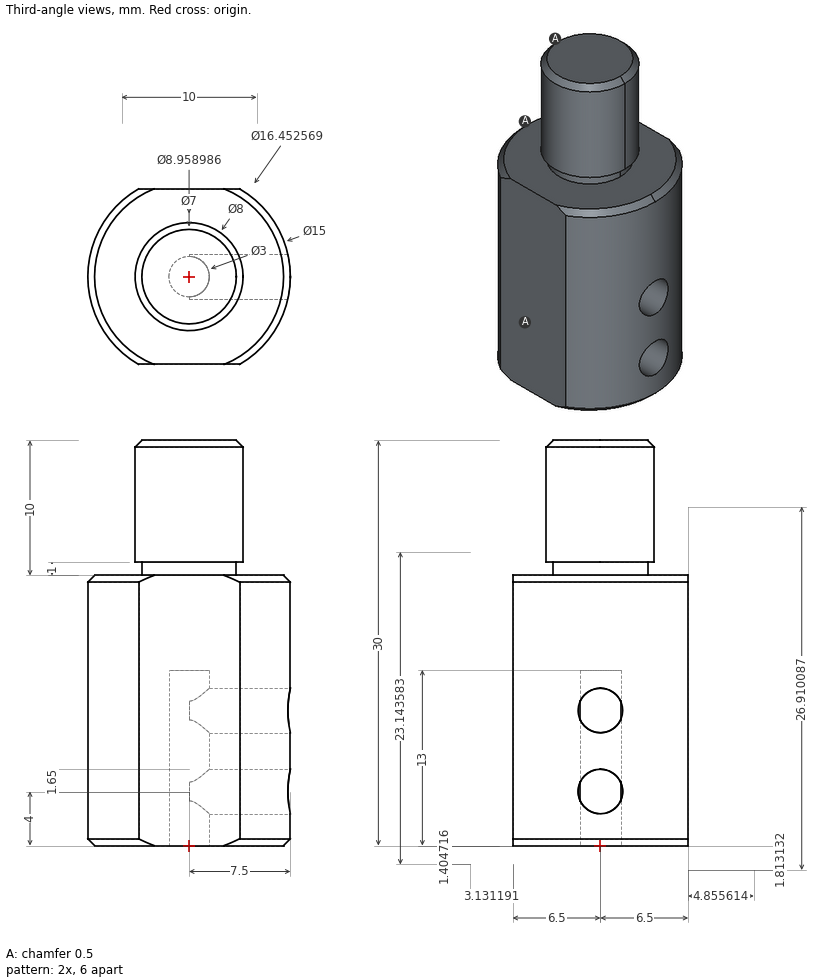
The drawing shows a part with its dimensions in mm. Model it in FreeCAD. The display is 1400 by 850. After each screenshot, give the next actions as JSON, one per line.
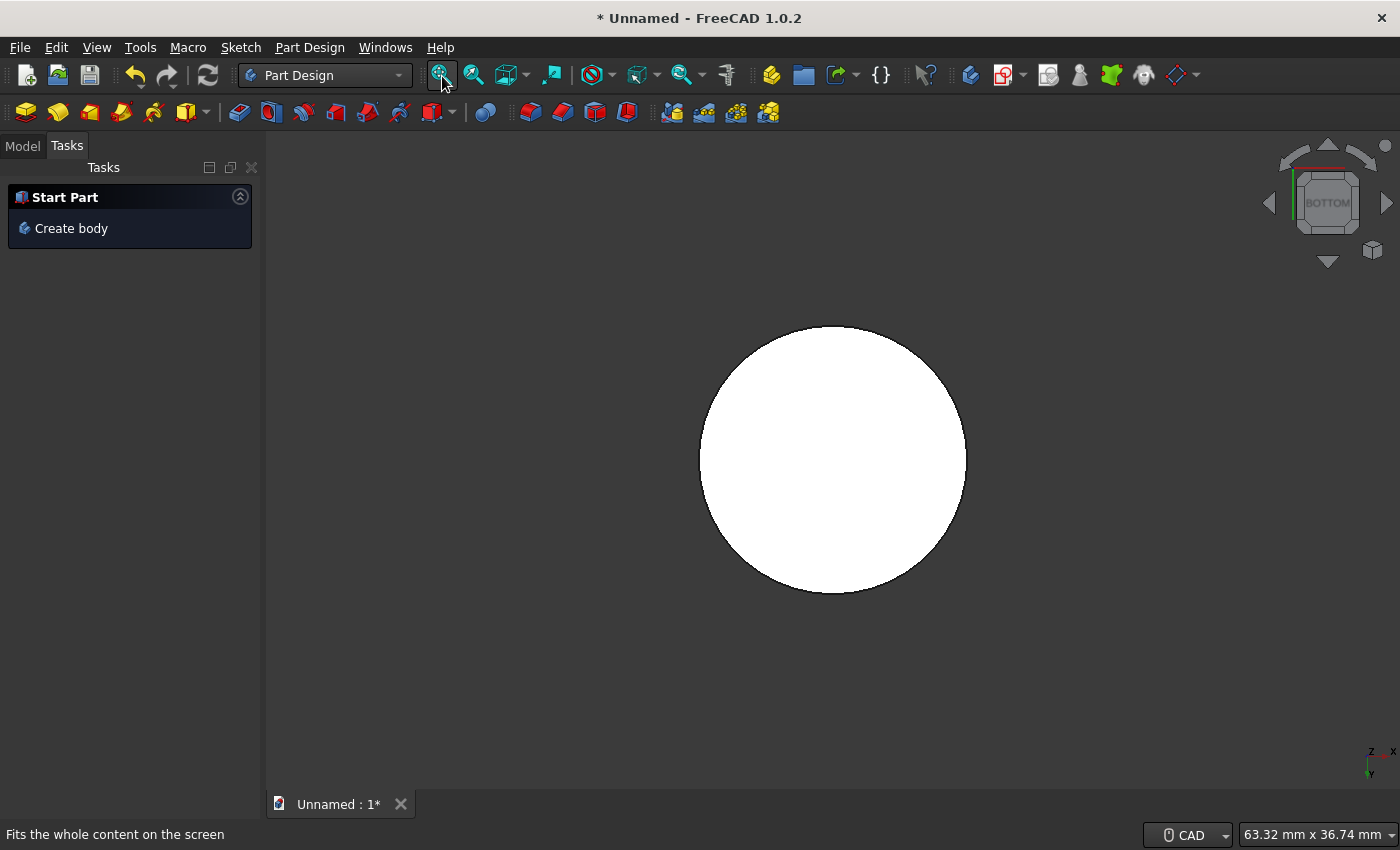
{"action": "left_click", "coordinate": [833, 459]}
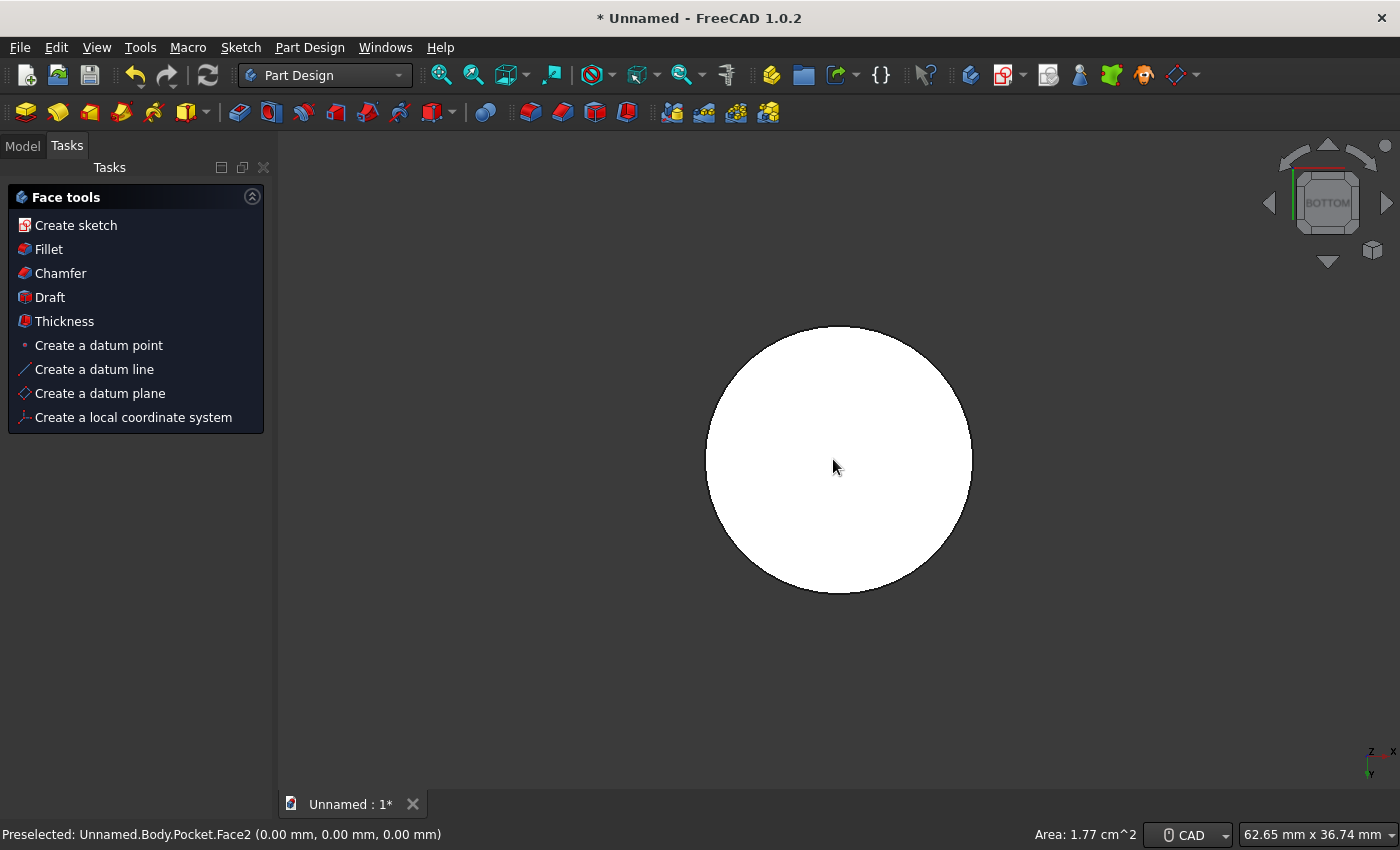
{"action": "left_click", "coordinate": [1004, 76]}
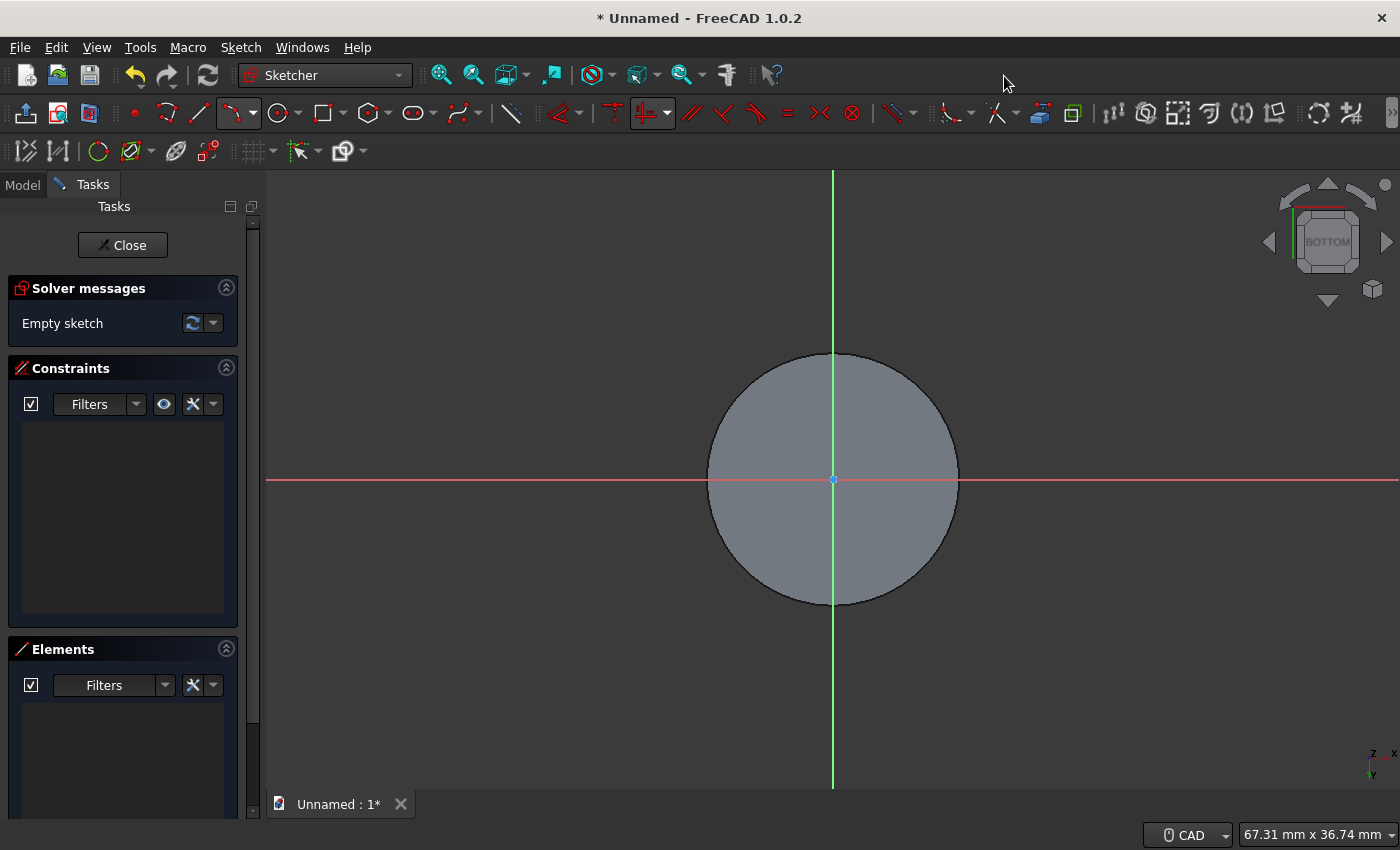
{"action": "scroll", "coordinate": [844, 480], "scroll_direction": "up", "scroll_amount": 10}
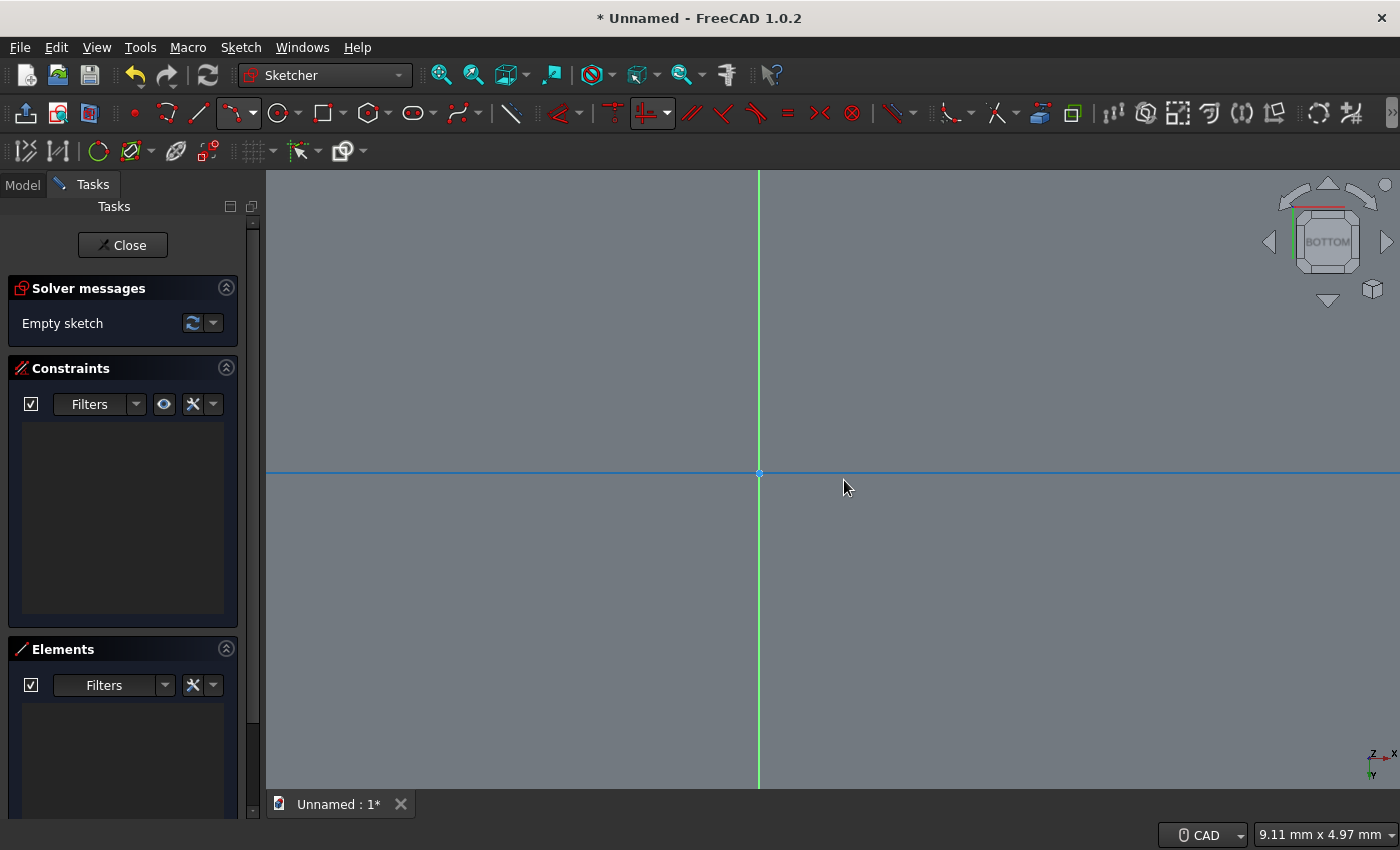
{"action": "left_click", "coordinate": [278, 114]}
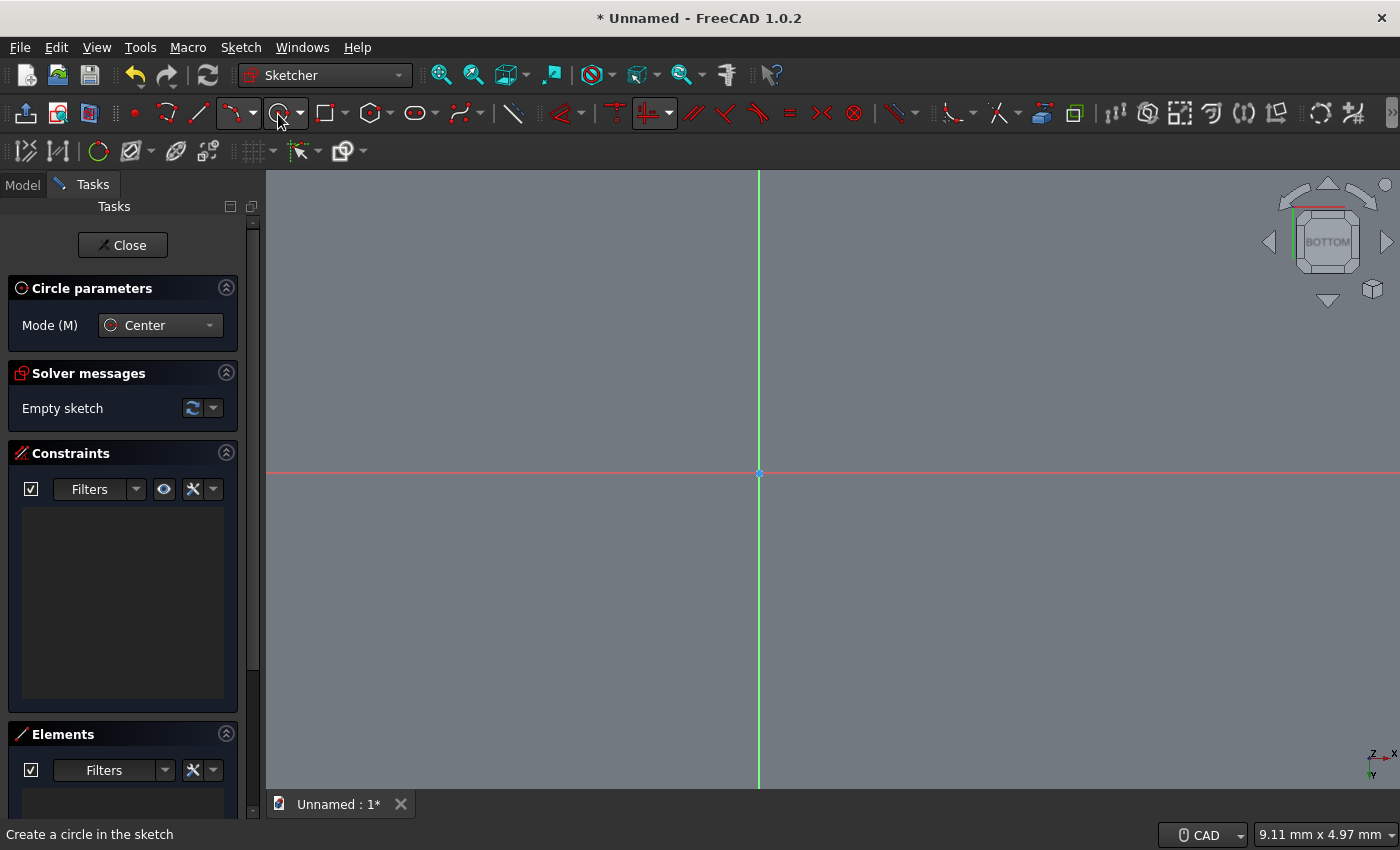
{"action": "left_click", "coordinate": [759, 473]}
{"action": "left_click", "coordinate": [891, 341]}
{"action": "key", "text": "Escape"}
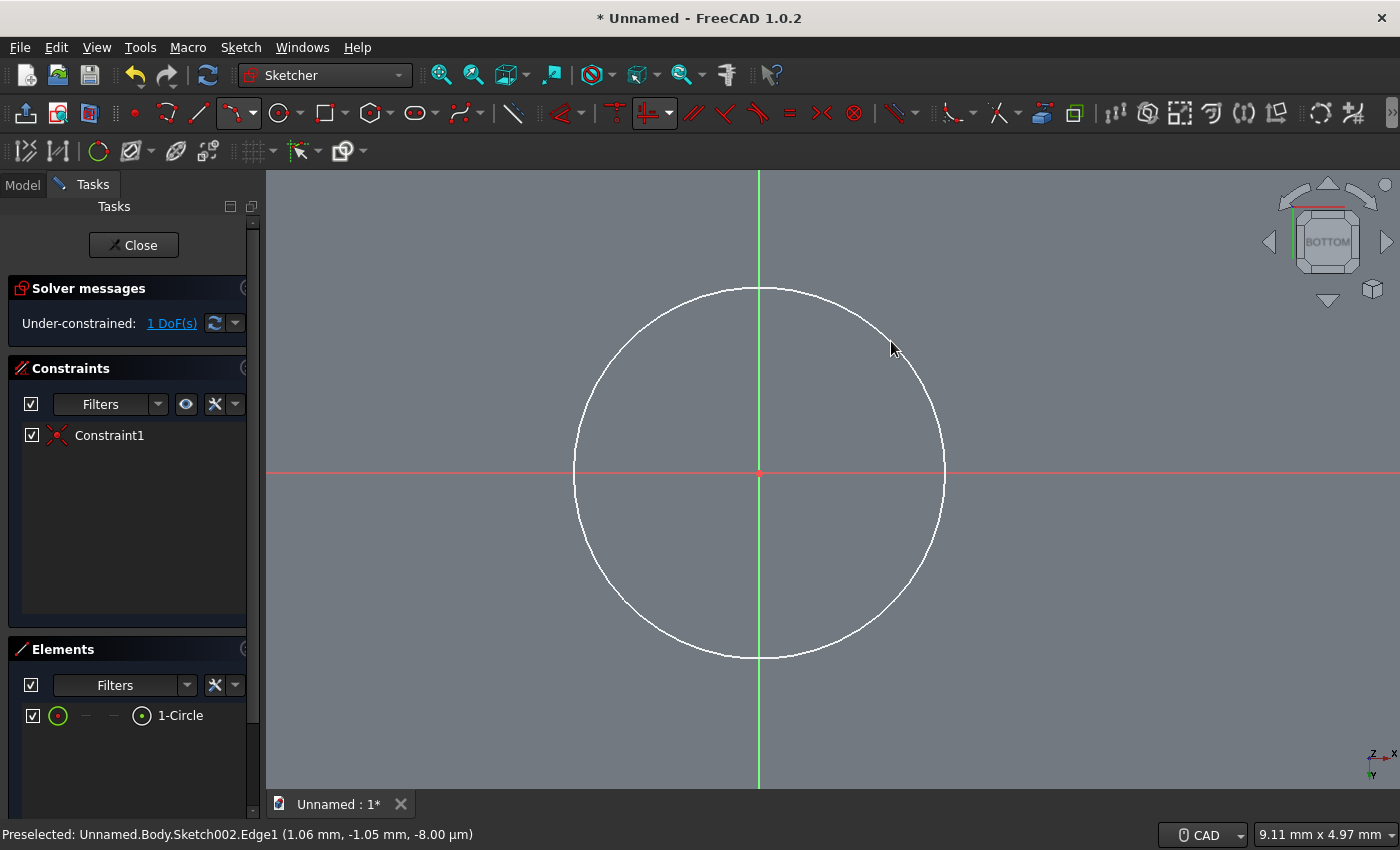
{"action": "left_click", "coordinate": [560, 114]}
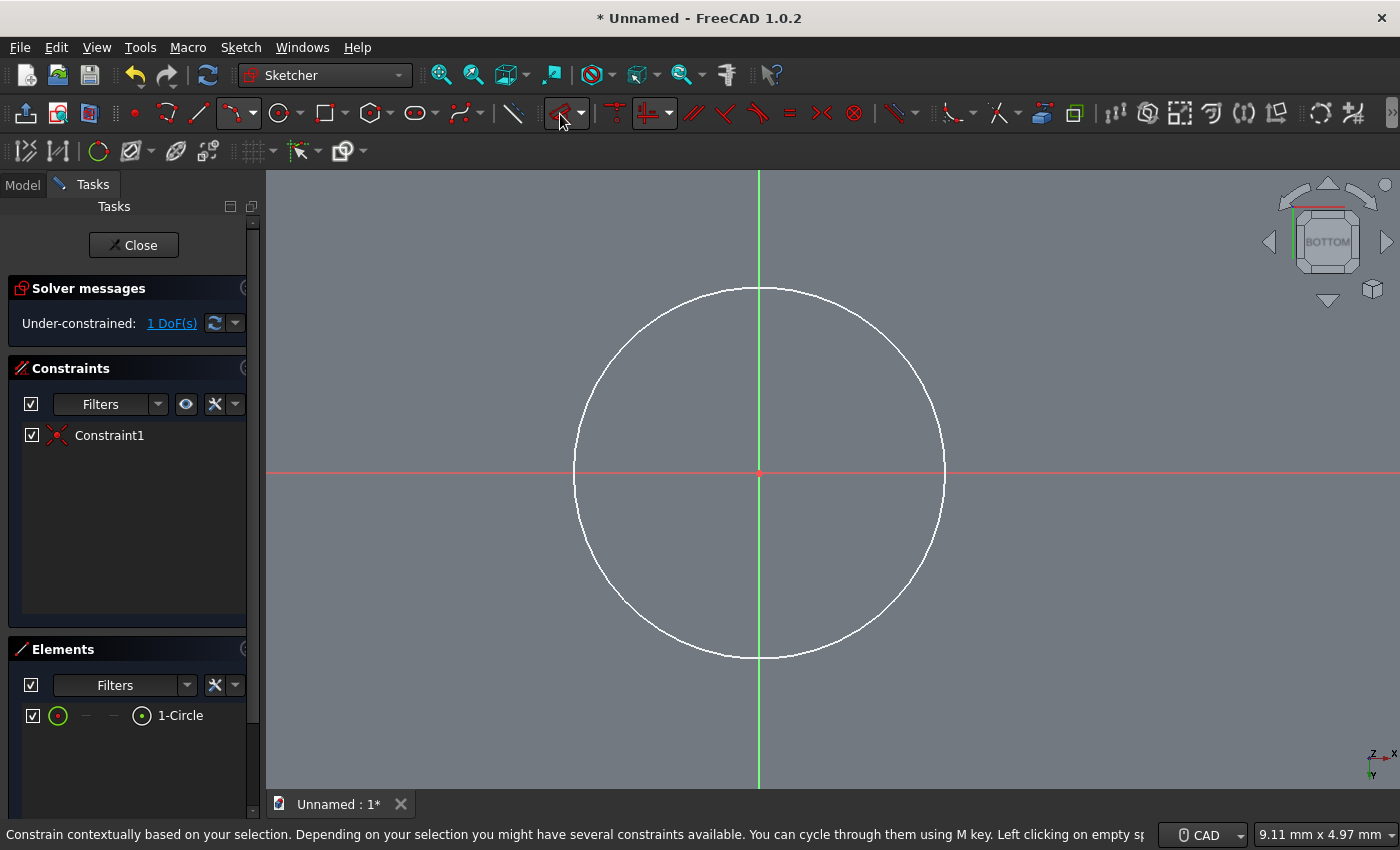
{"action": "left_click", "coordinate": [890, 341]}
{"action": "left_click", "coordinate": [912, 318]}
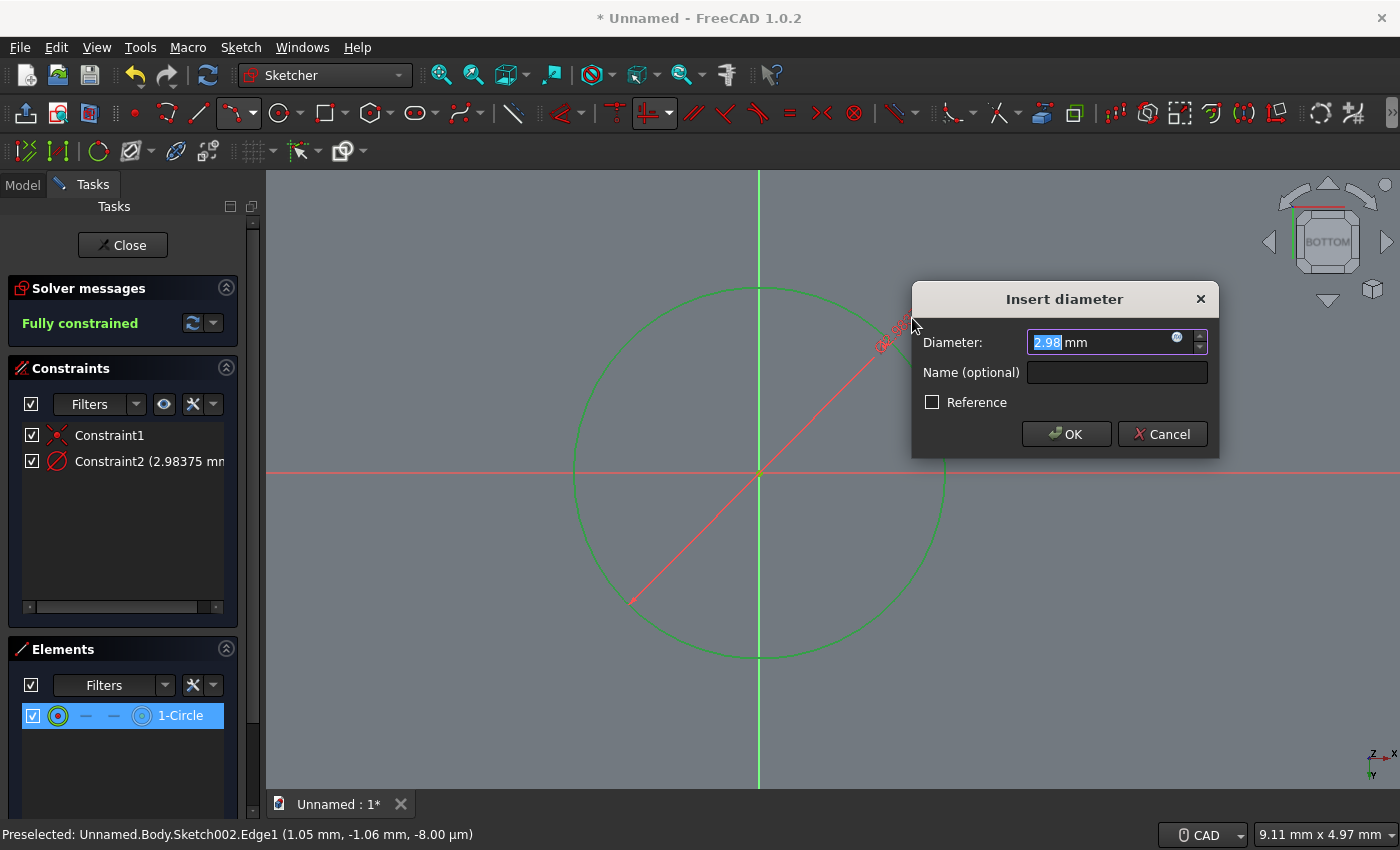
{"action": "type", "text": "3"}
{"action": "key", "text": "Return"}
{"action": "key", "text": "Escape"}